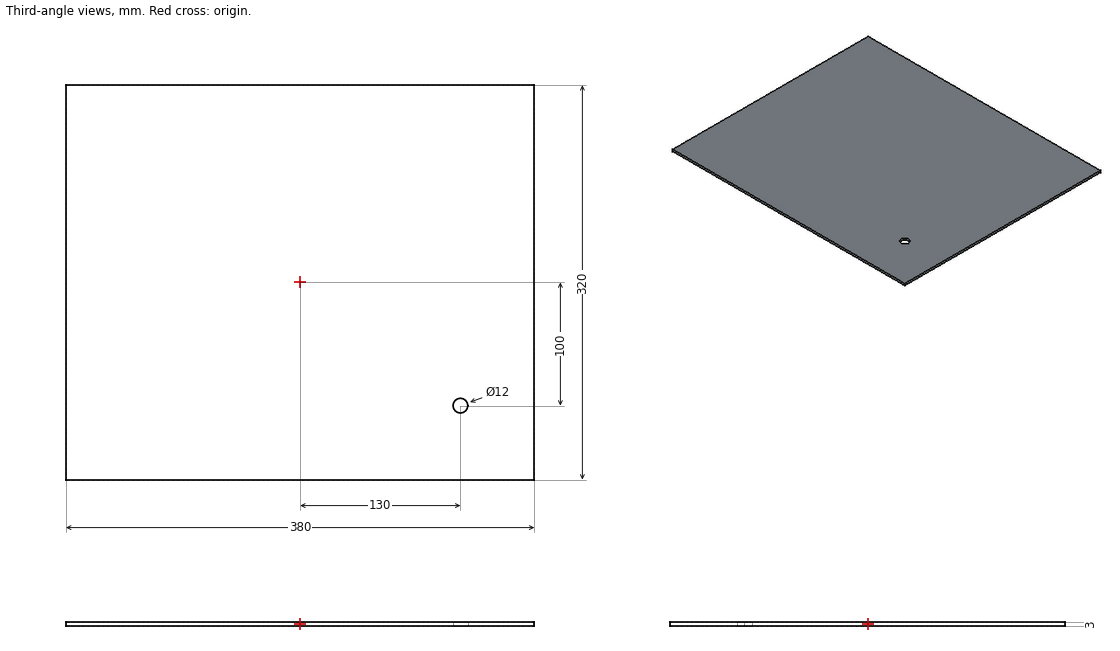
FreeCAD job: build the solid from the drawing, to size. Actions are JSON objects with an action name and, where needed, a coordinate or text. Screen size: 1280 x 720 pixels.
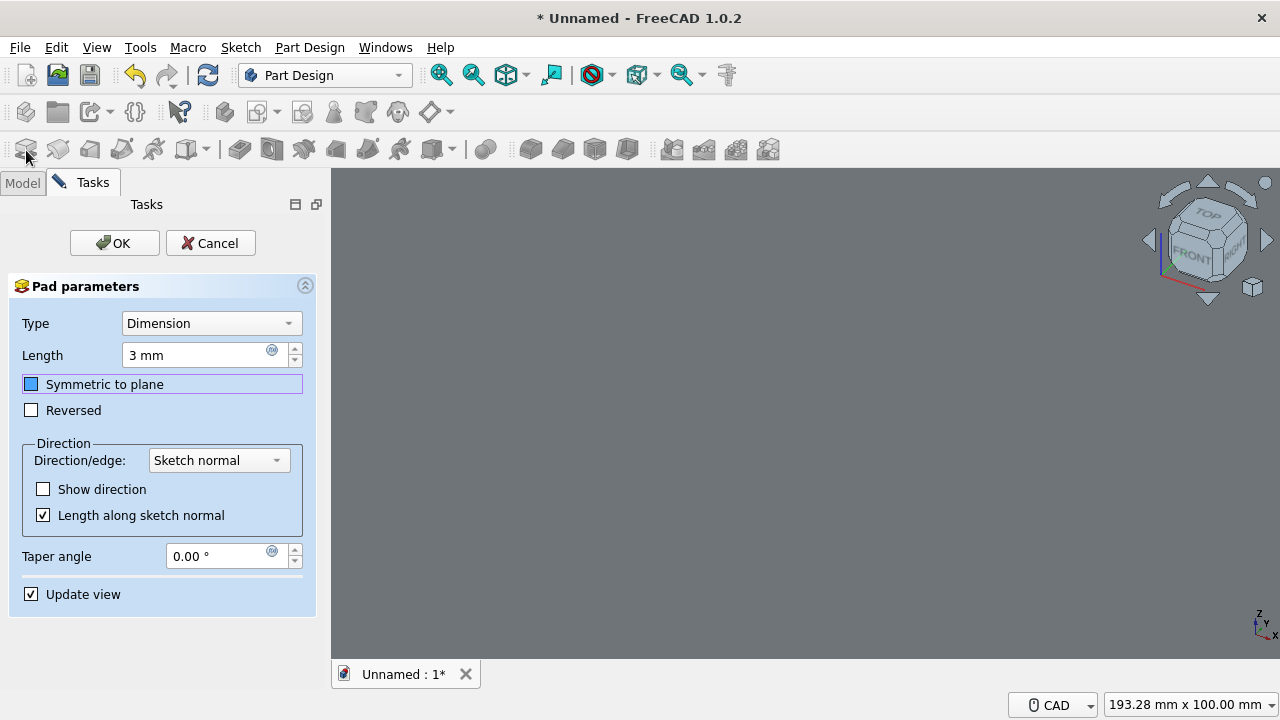
{"action": "left_click", "coordinate": [30, 384]}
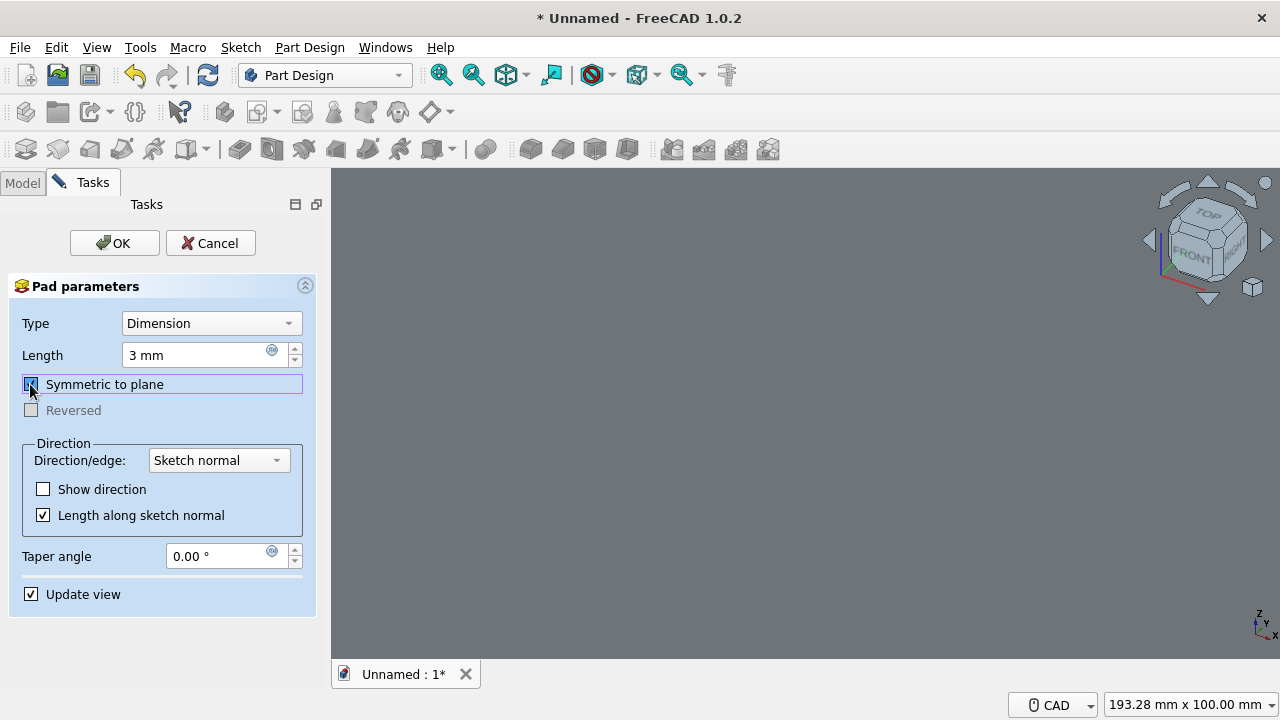
{"action": "left_click", "coordinate": [115, 243]}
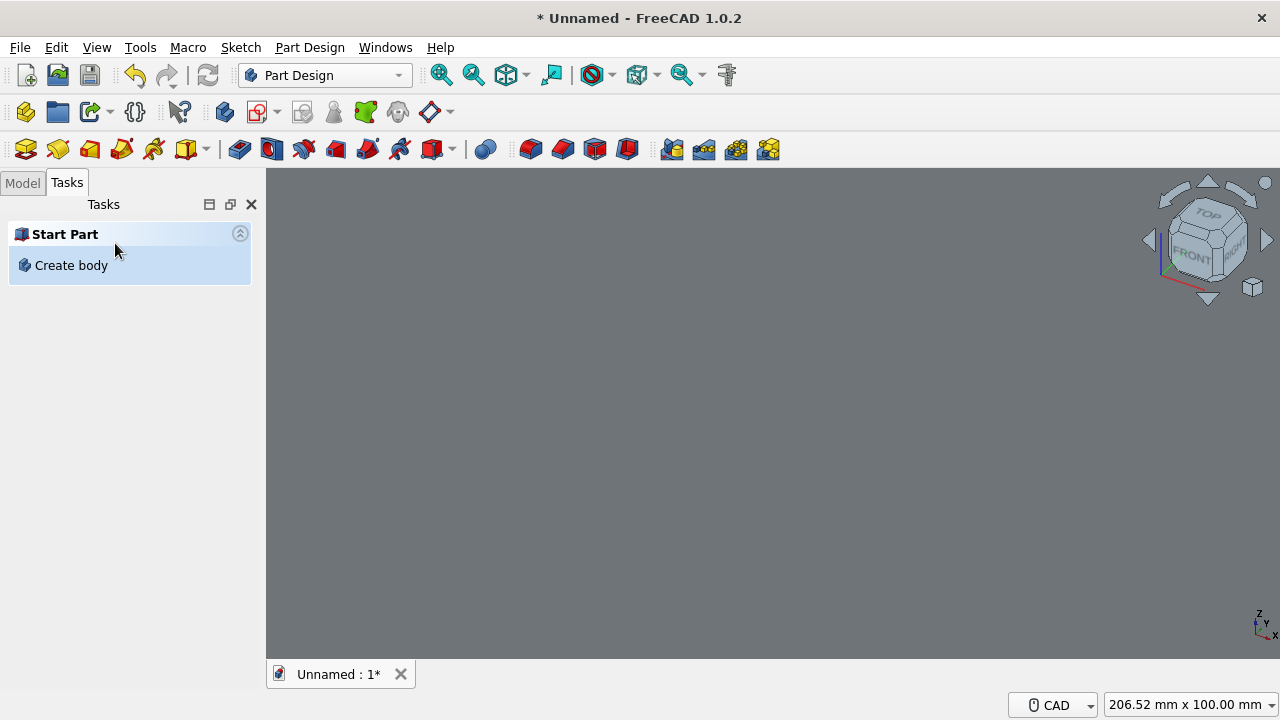
{"action": "left_click", "coordinate": [442, 76]}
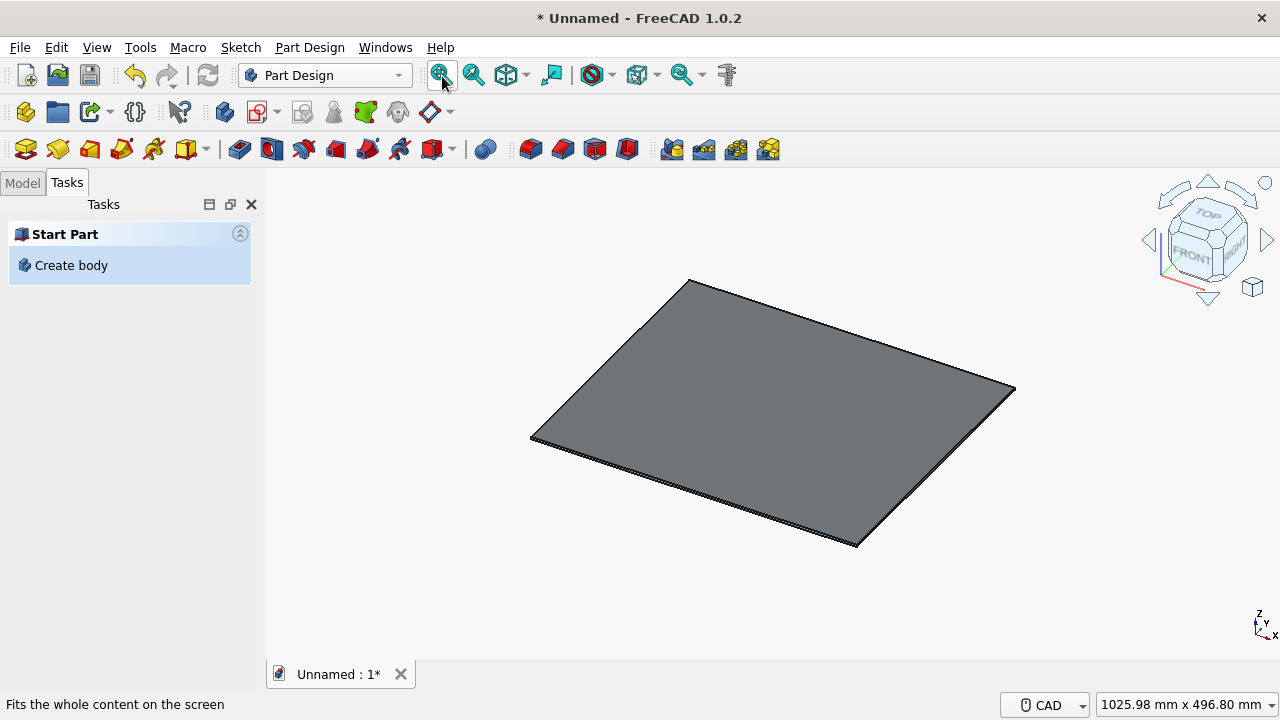
{"action": "left_click", "coordinate": [258, 112]}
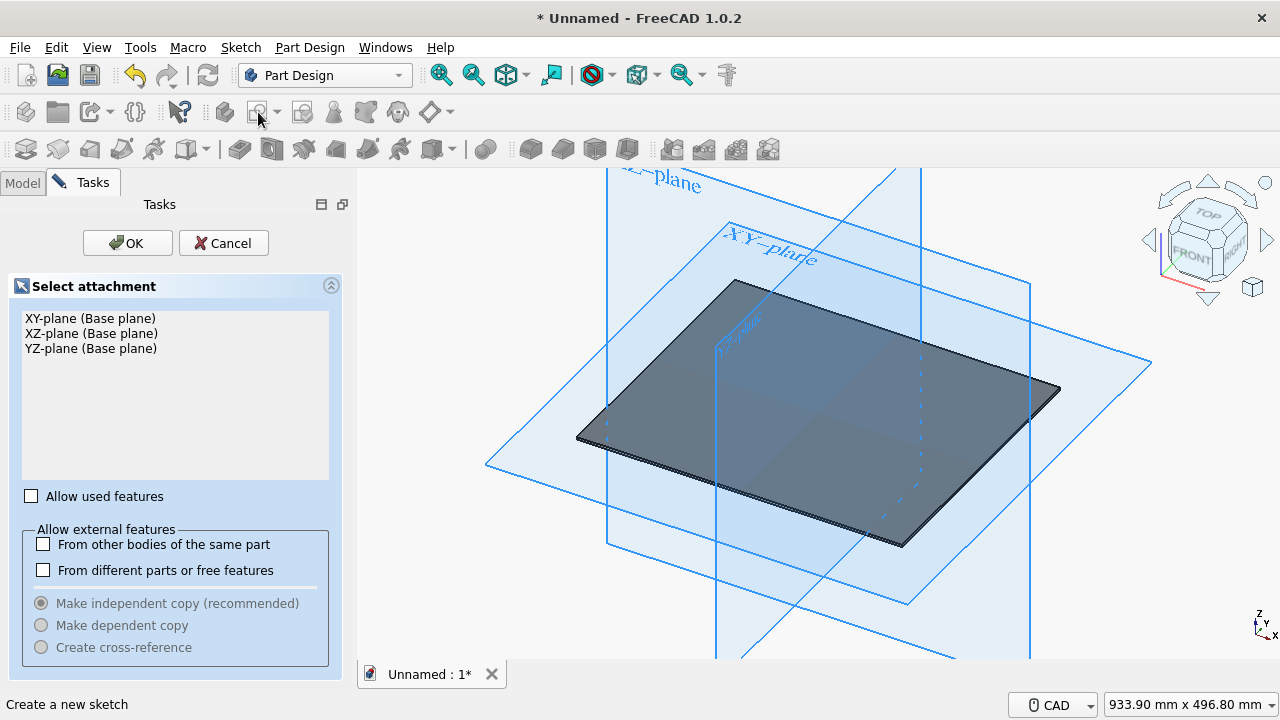
{"action": "left_click", "coordinate": [82, 318]}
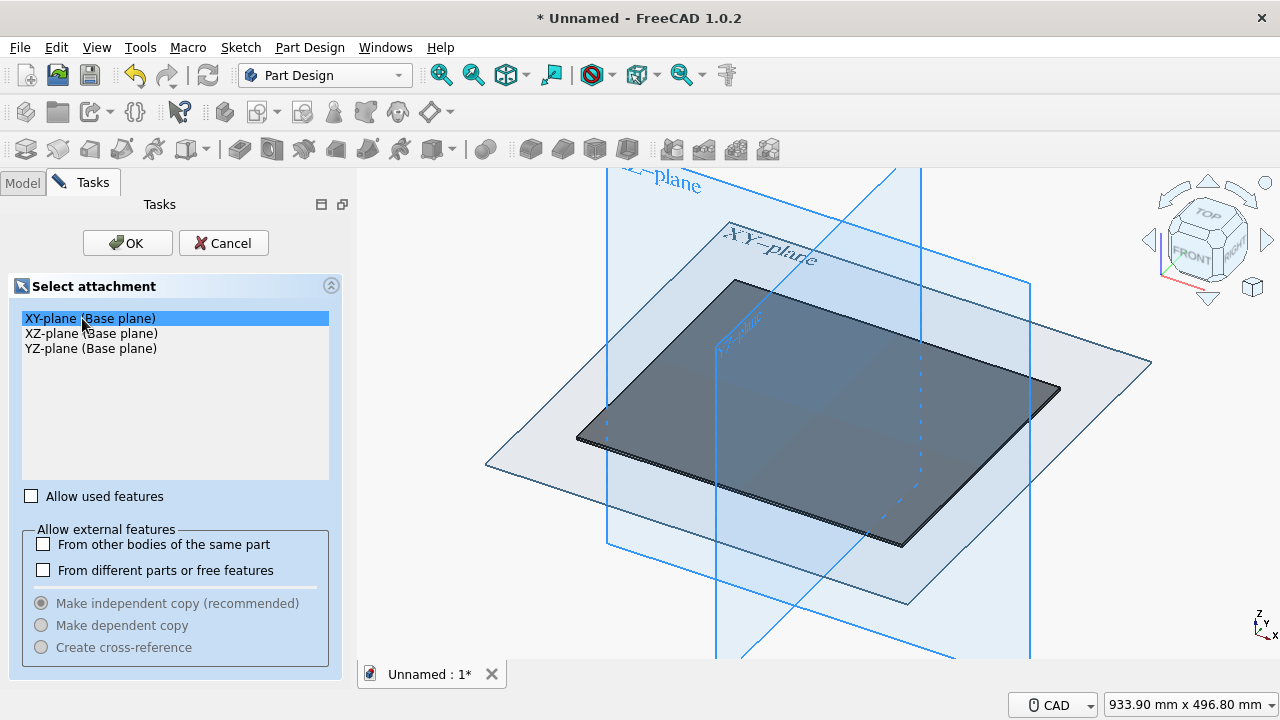
{"action": "left_click", "coordinate": [128, 243]}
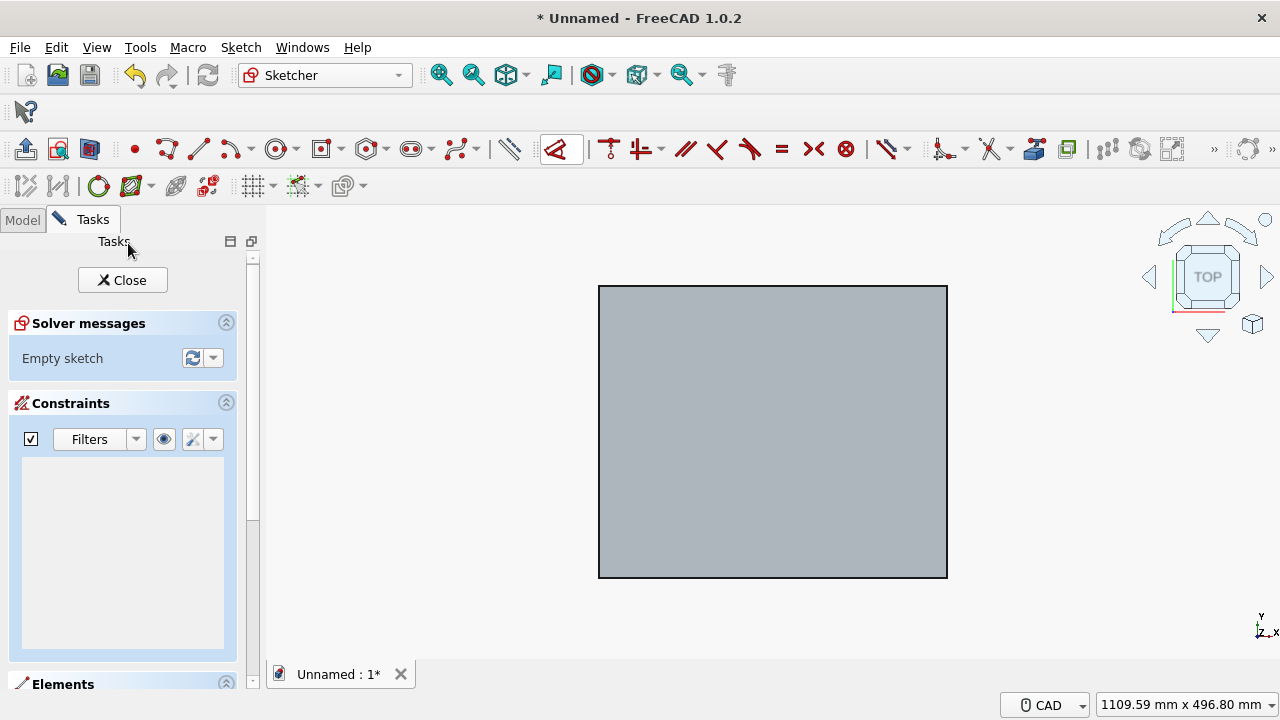
{"action": "left_click", "coordinate": [90, 150]}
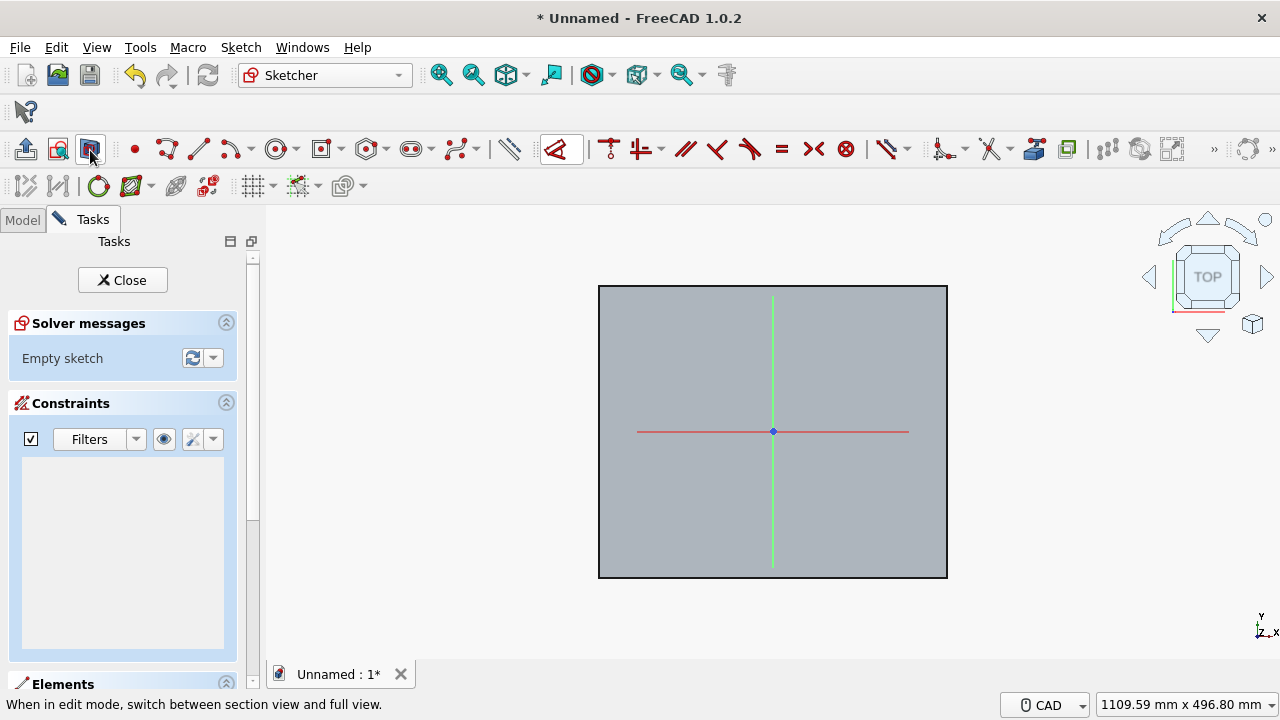
{"action": "scroll", "coordinate": [902, 528], "scroll_direction": "up", "scroll_amount": 15}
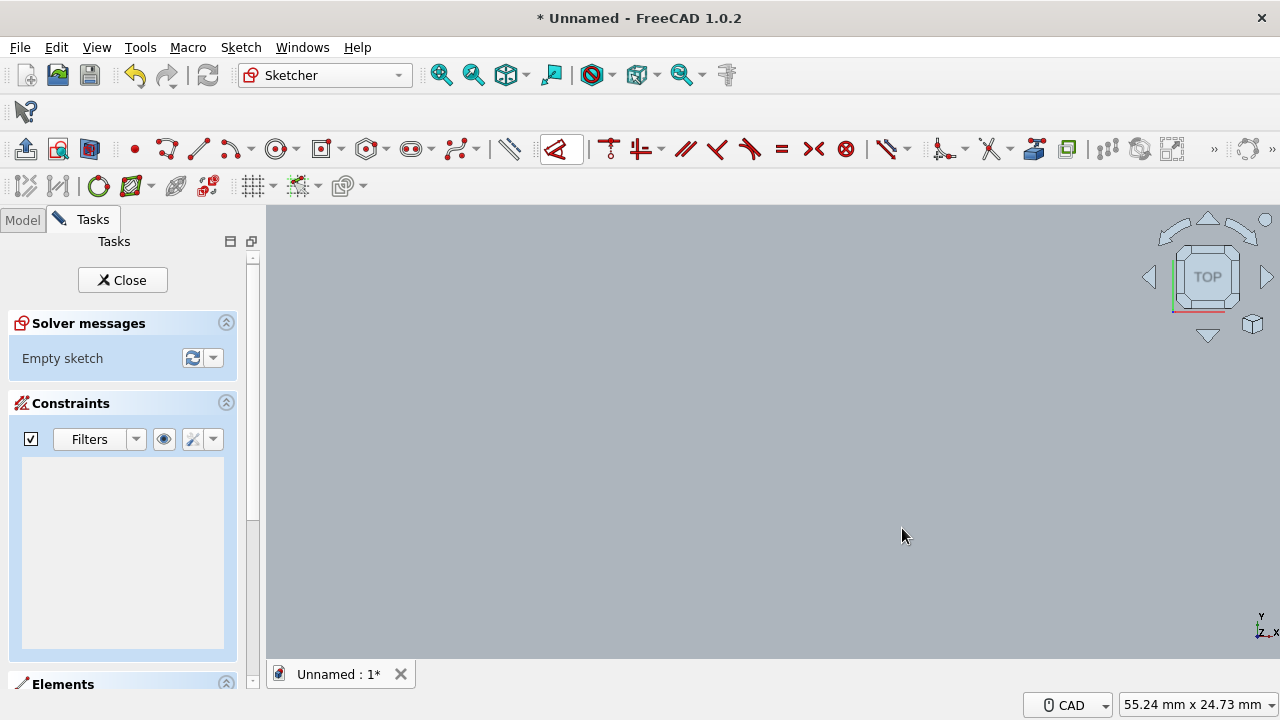
{"action": "left_click", "coordinate": [276, 150]}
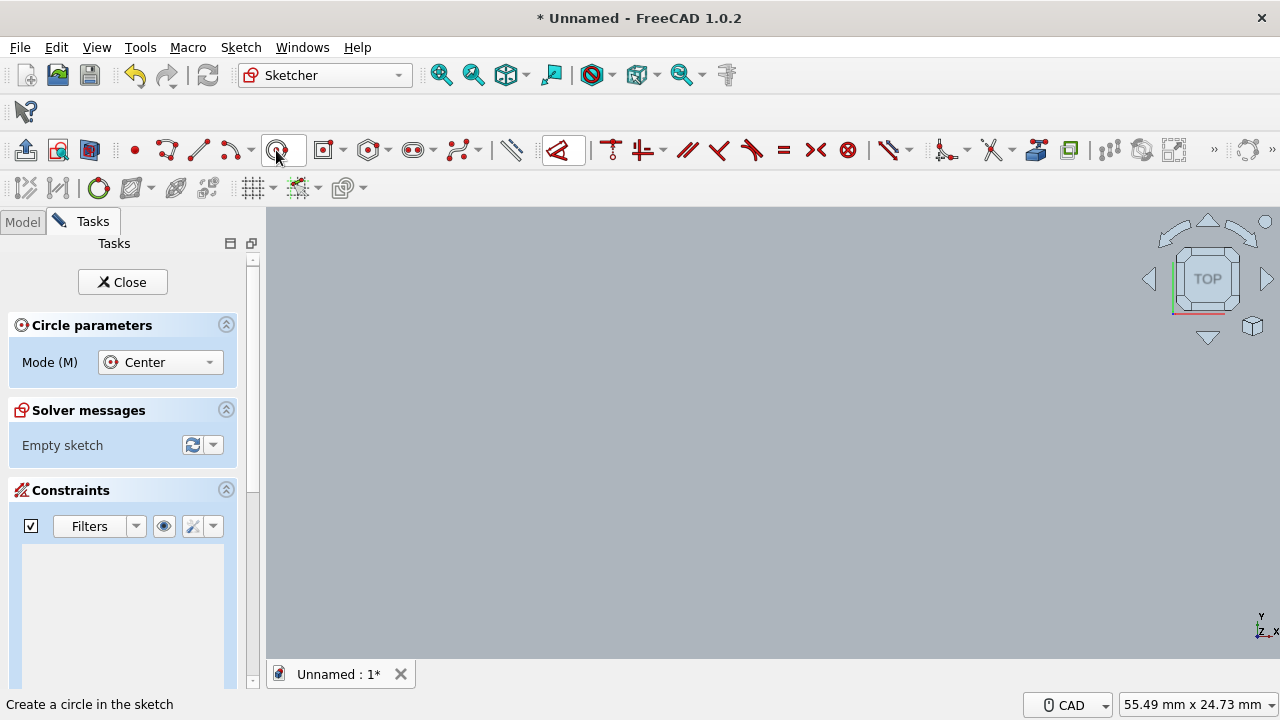
{"action": "left_click", "coordinate": [686, 423]}
{"action": "mouse_move", "coordinate": [763, 345]}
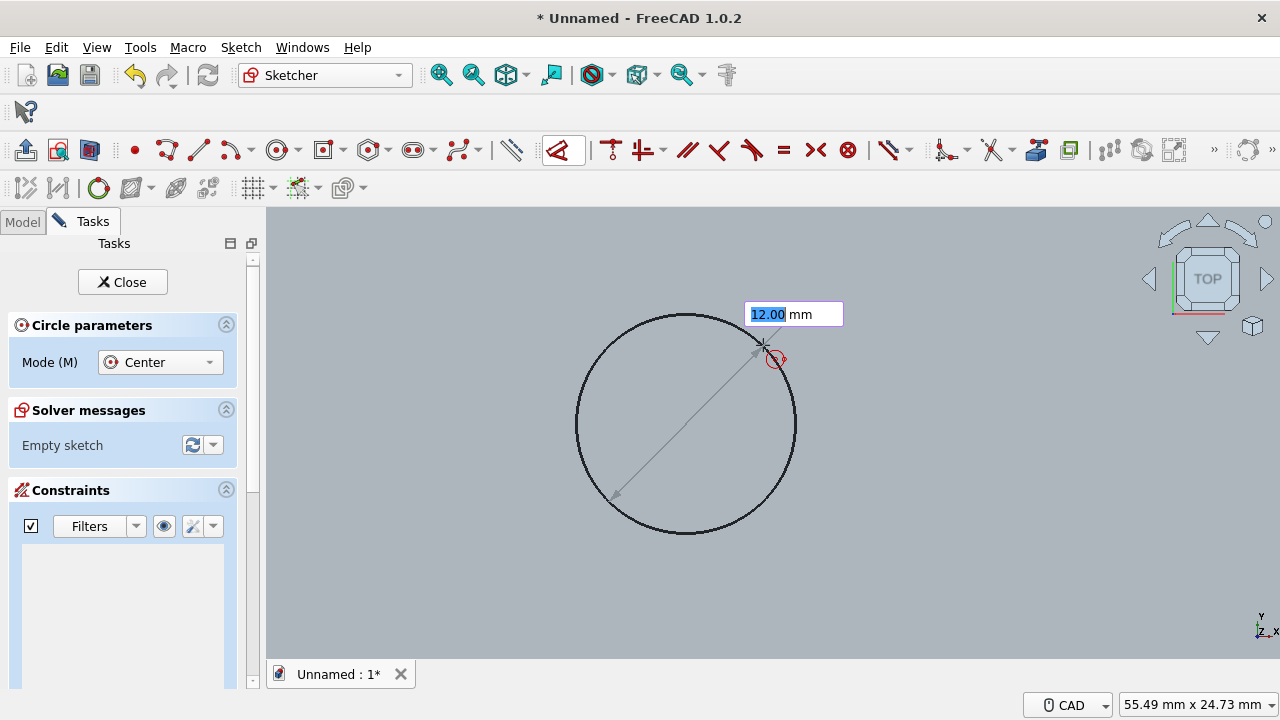
{"action": "type", "text": "12"}
{"action": "key", "text": "Return"}
{"action": "key", "text": "Escape"}